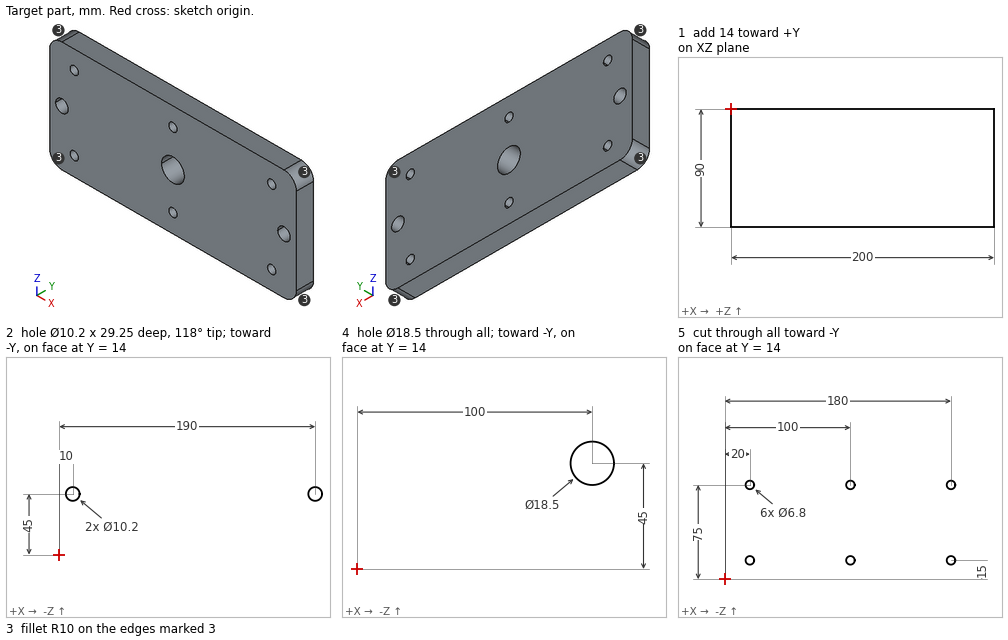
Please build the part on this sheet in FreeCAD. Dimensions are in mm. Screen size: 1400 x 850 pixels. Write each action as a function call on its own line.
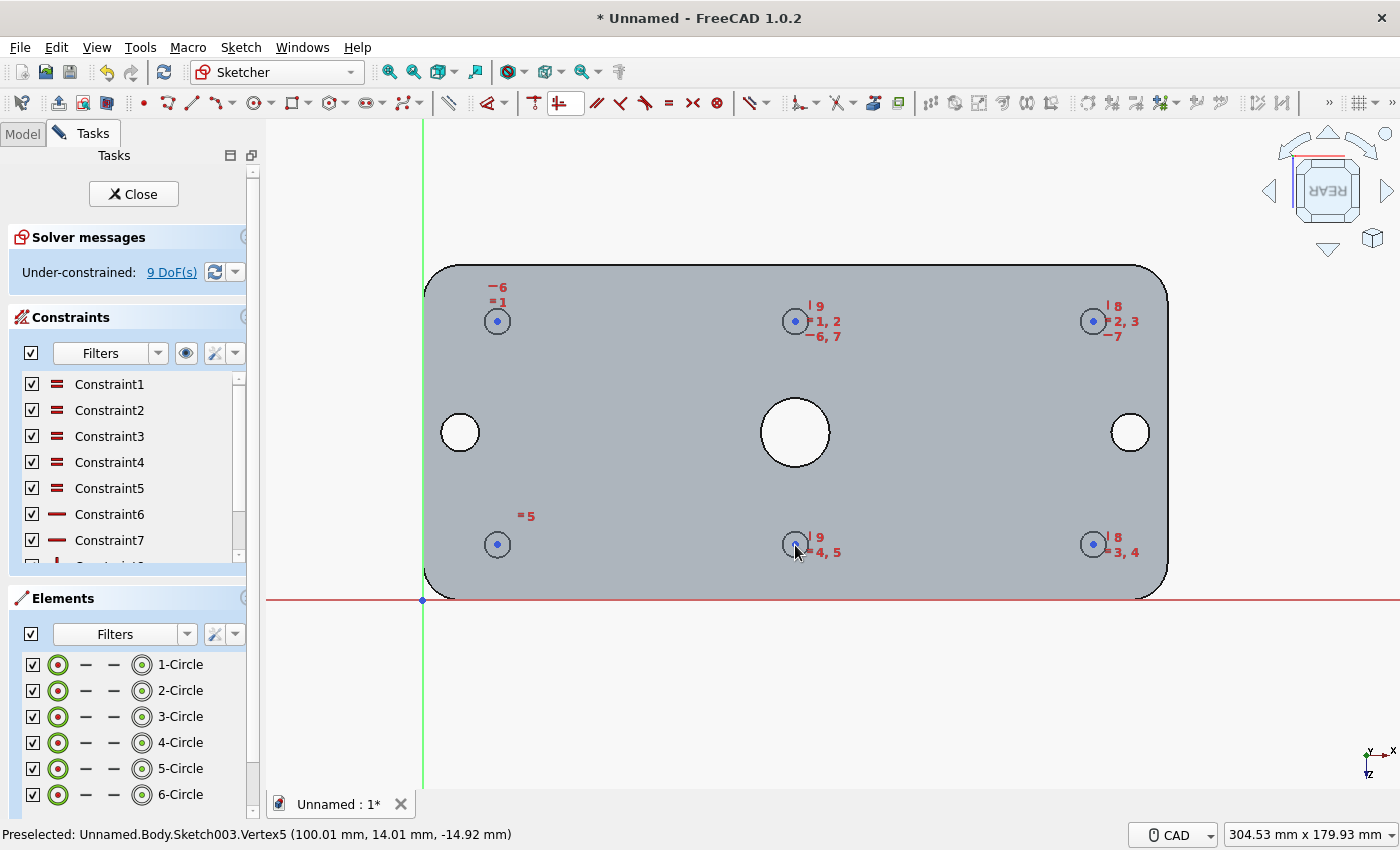
click(1093, 545)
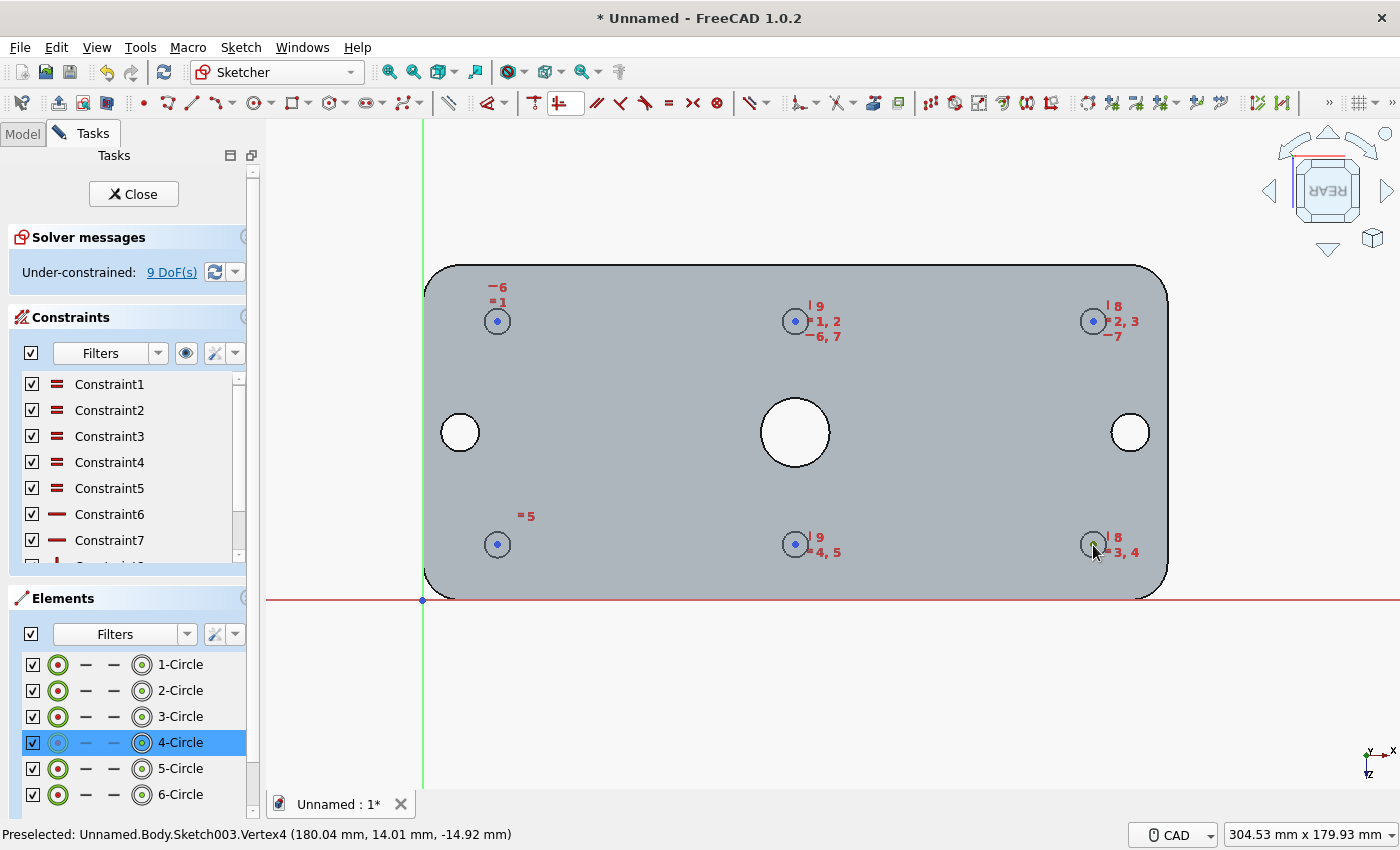
click(795, 545)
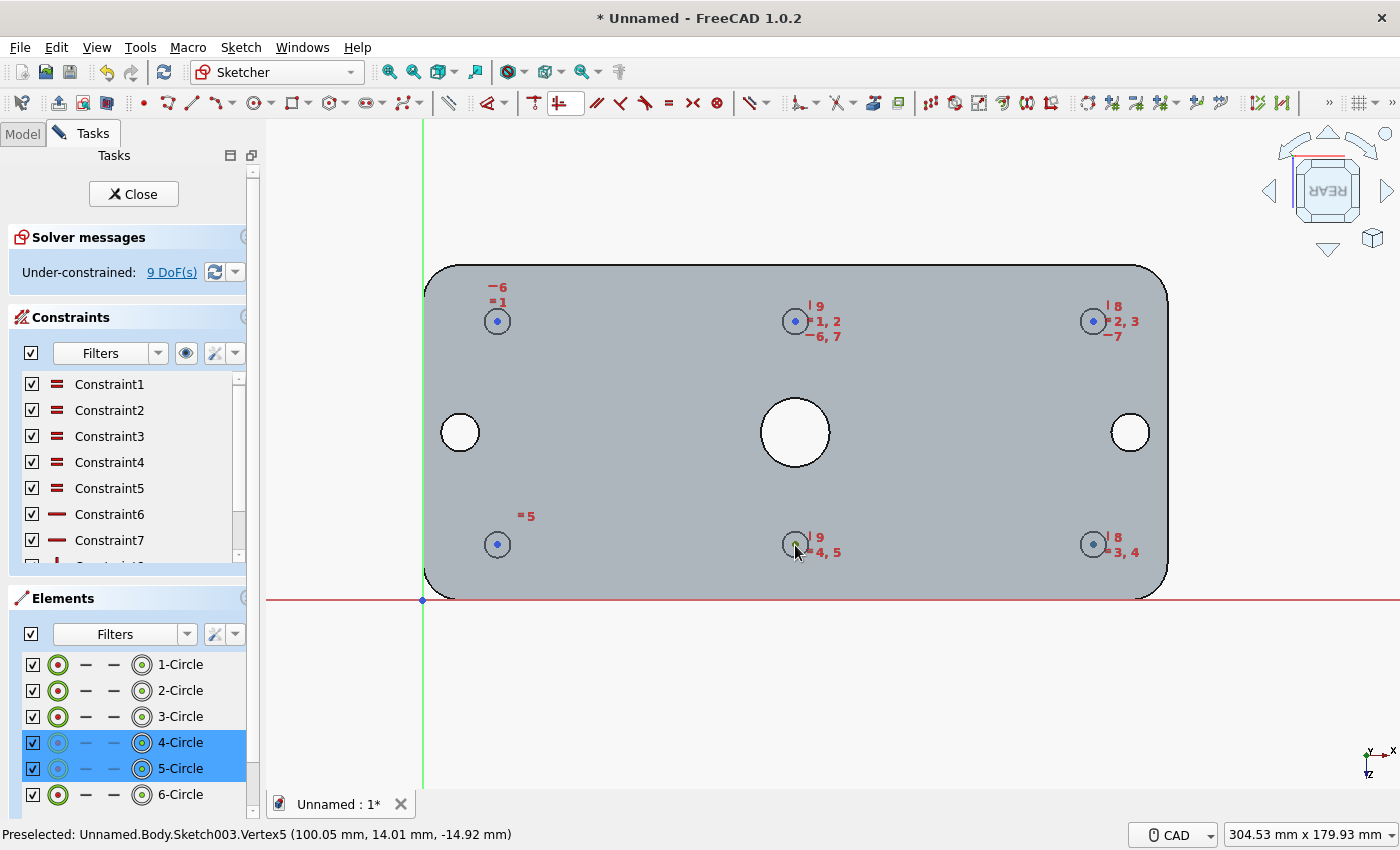
key(h)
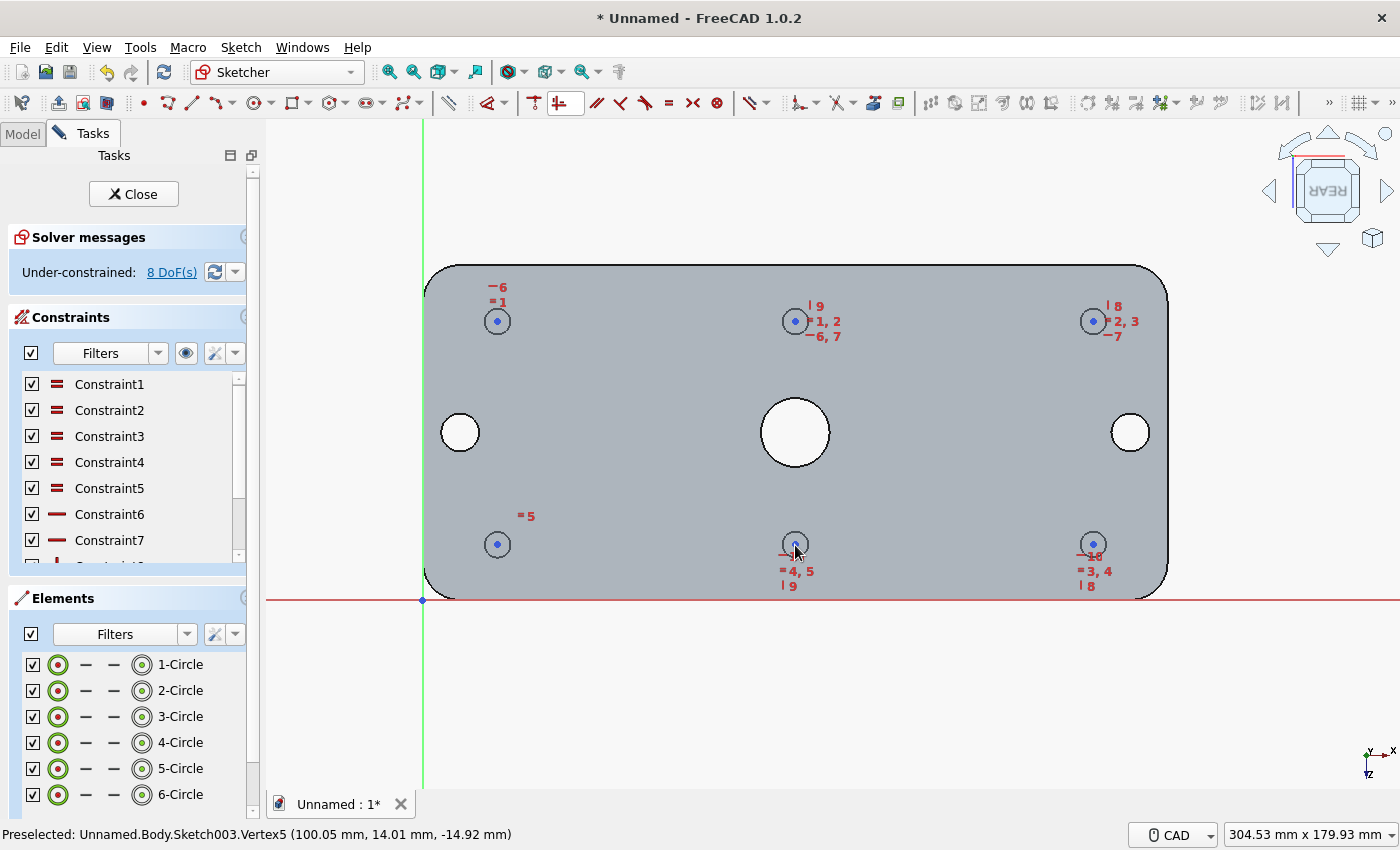
click(497, 322)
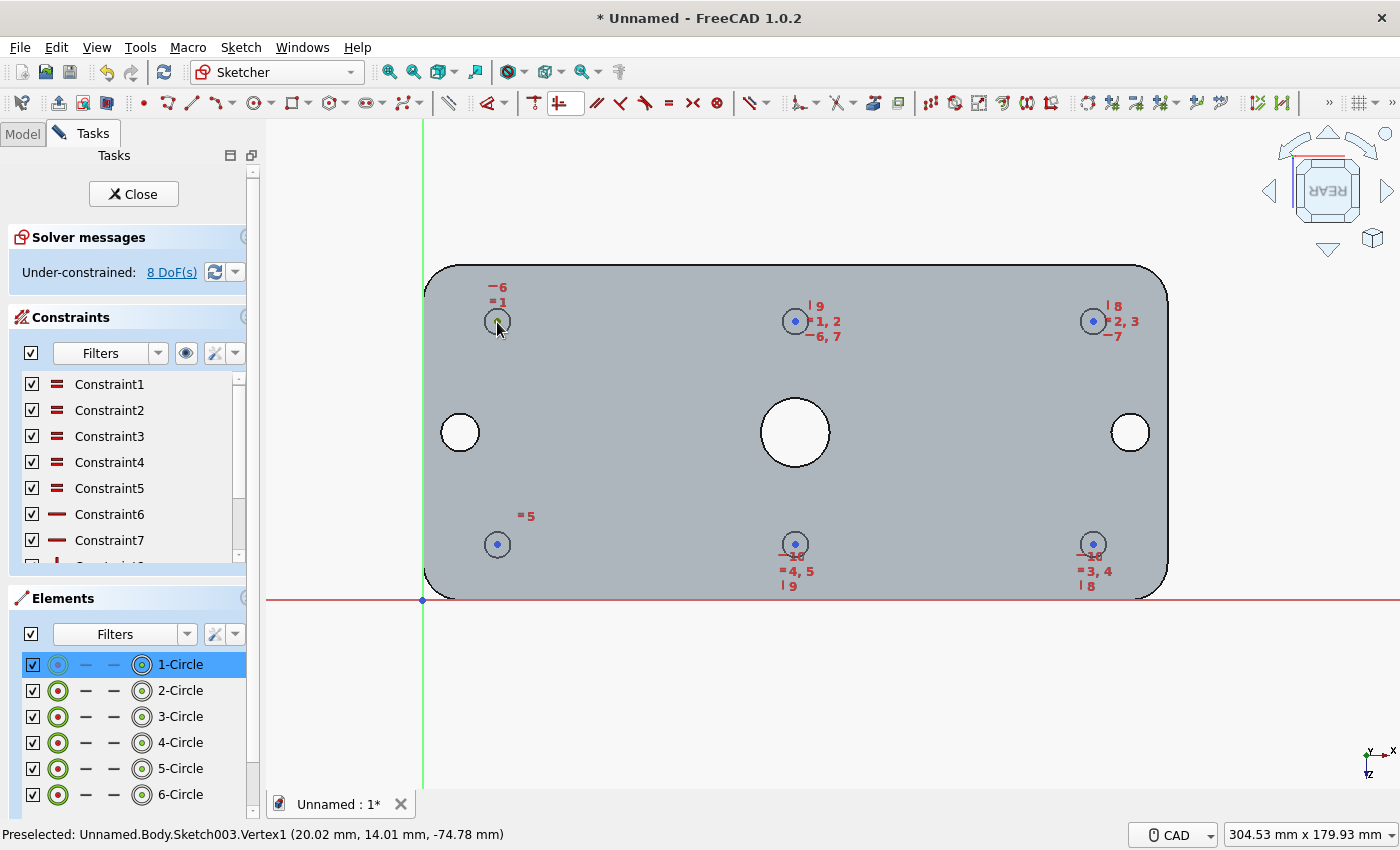
click(498, 545)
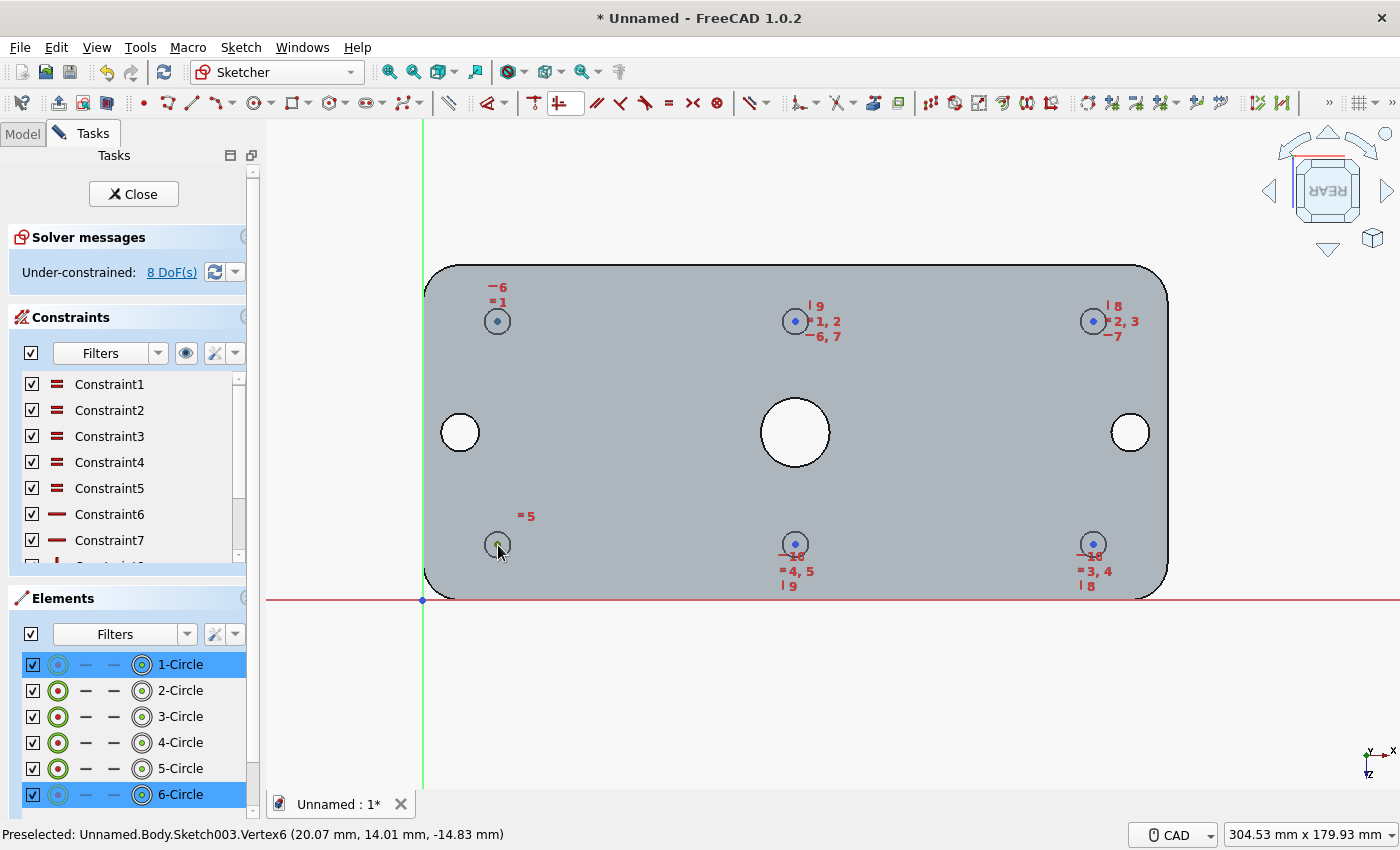
click(578, 104)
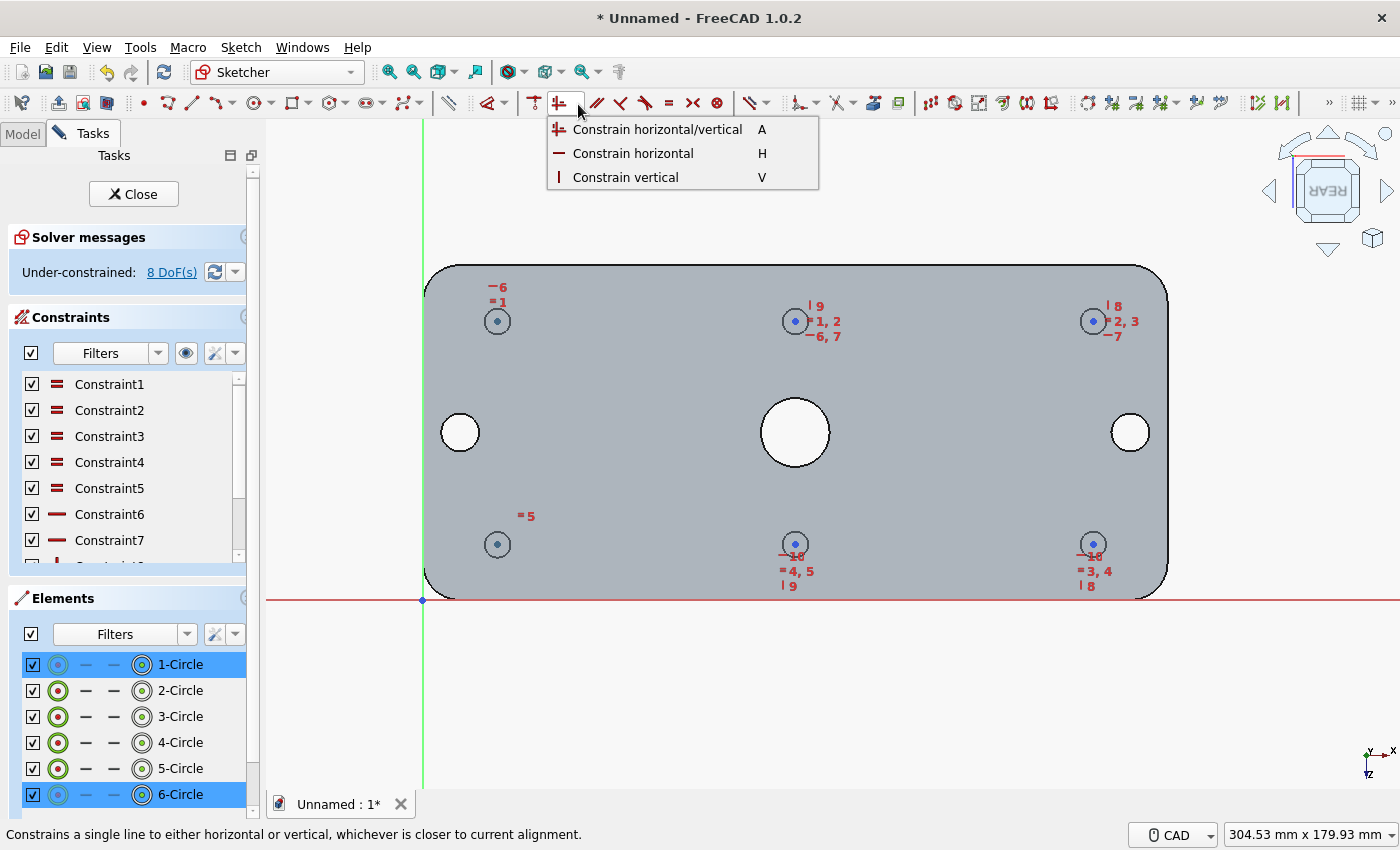
click(683, 177)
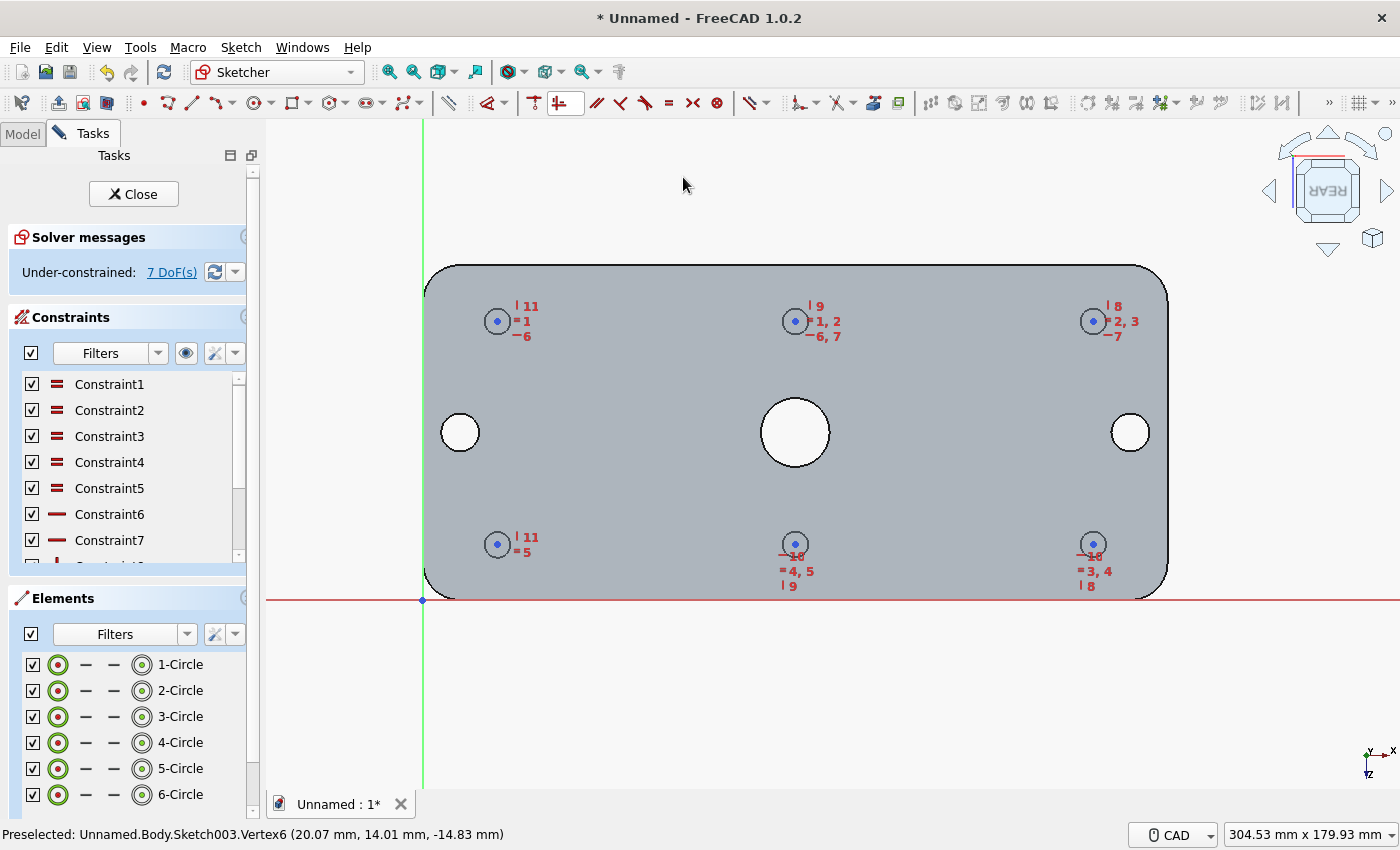
click(795, 545)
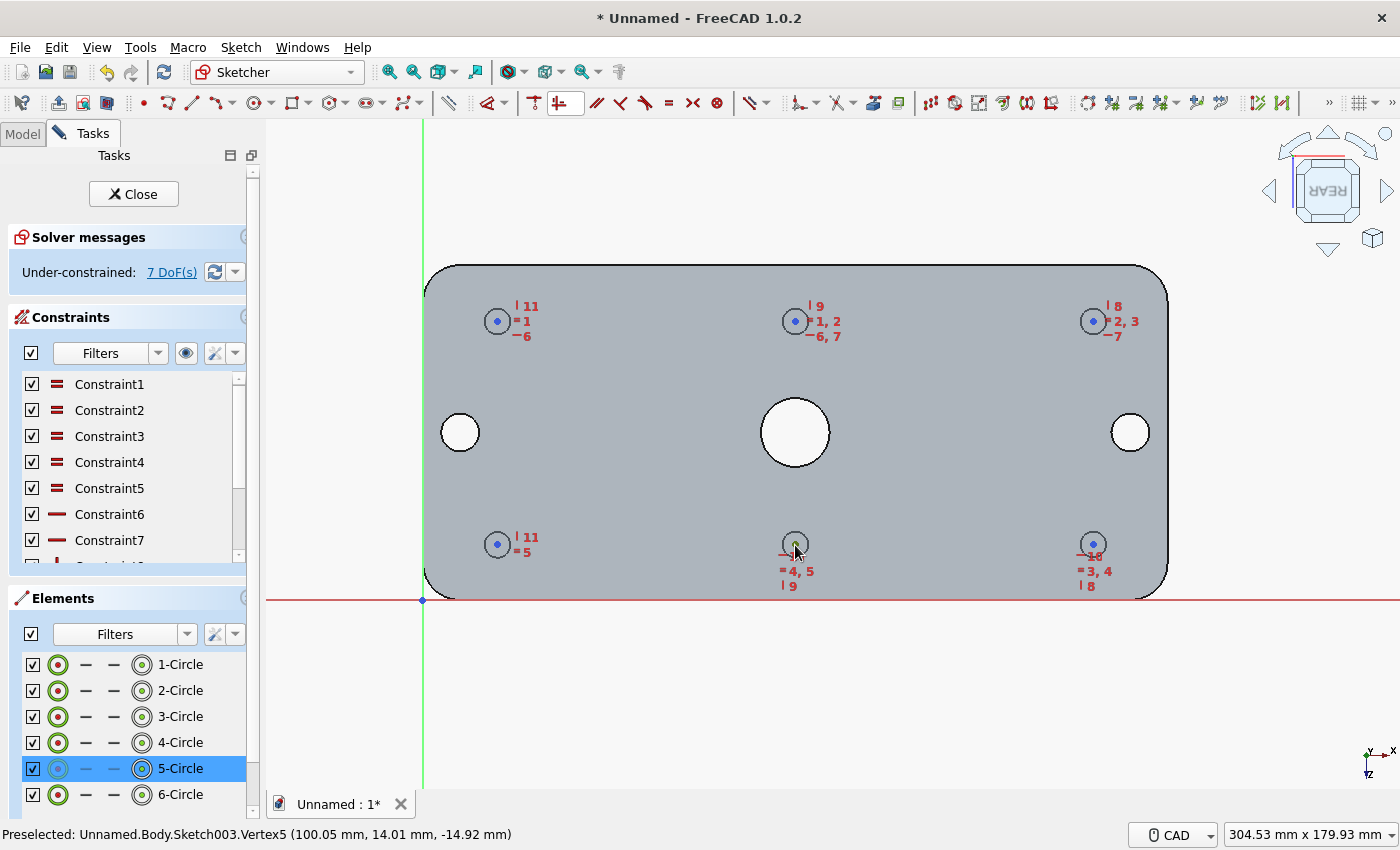
click(497, 545)